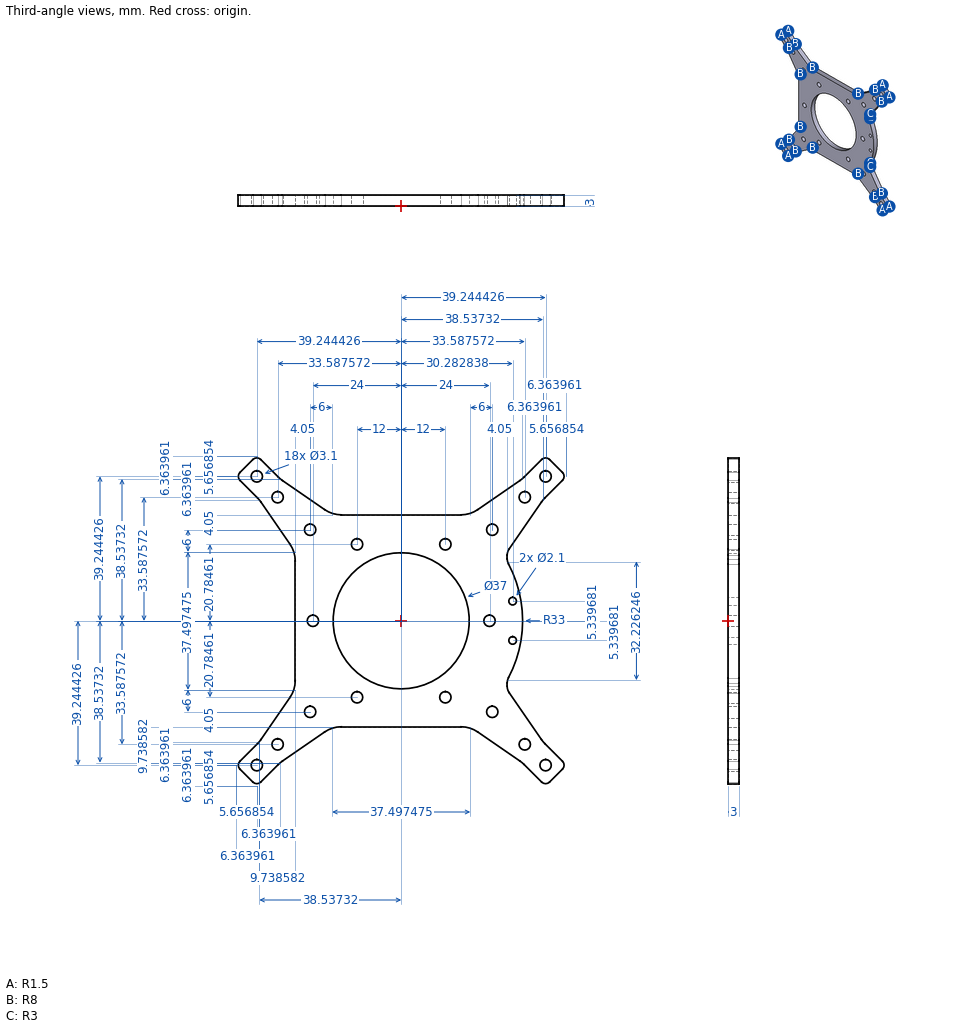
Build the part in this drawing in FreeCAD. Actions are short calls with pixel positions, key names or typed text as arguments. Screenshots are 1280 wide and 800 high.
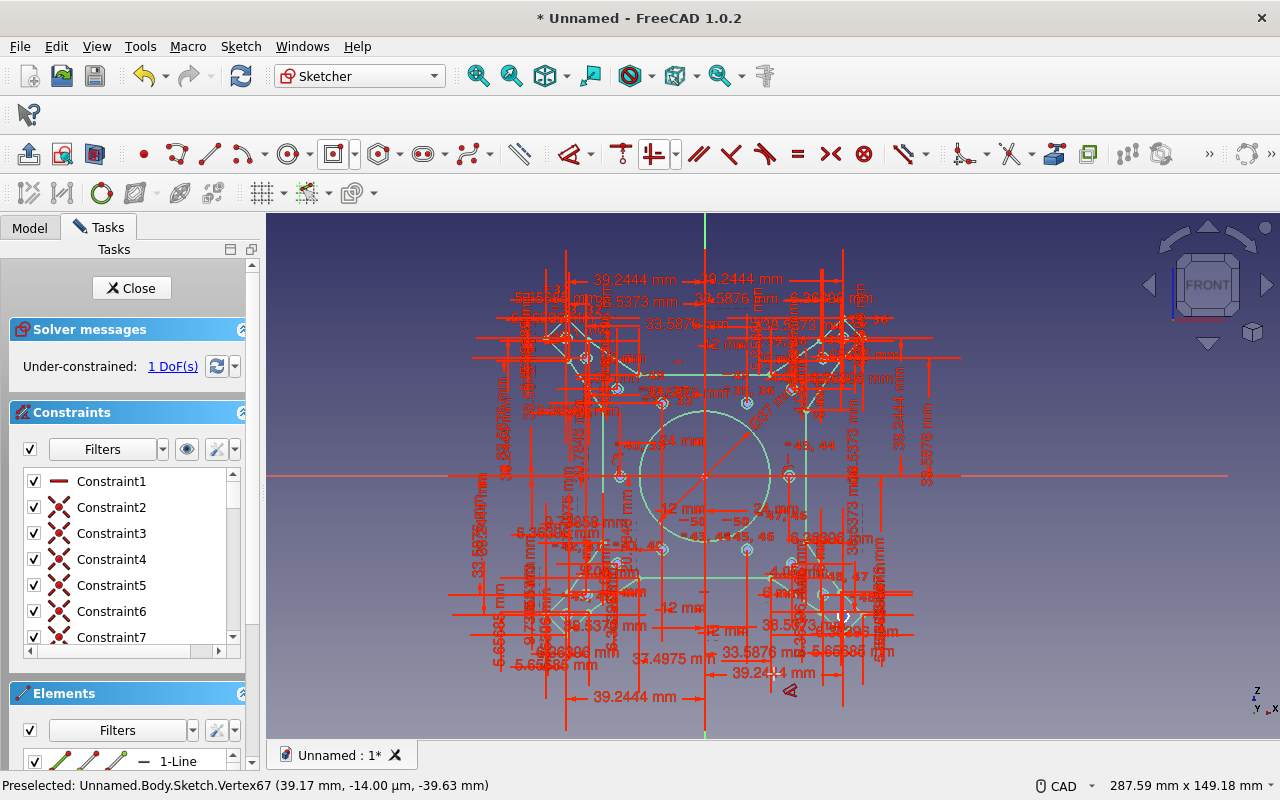
click(843, 616)
click(925, 546)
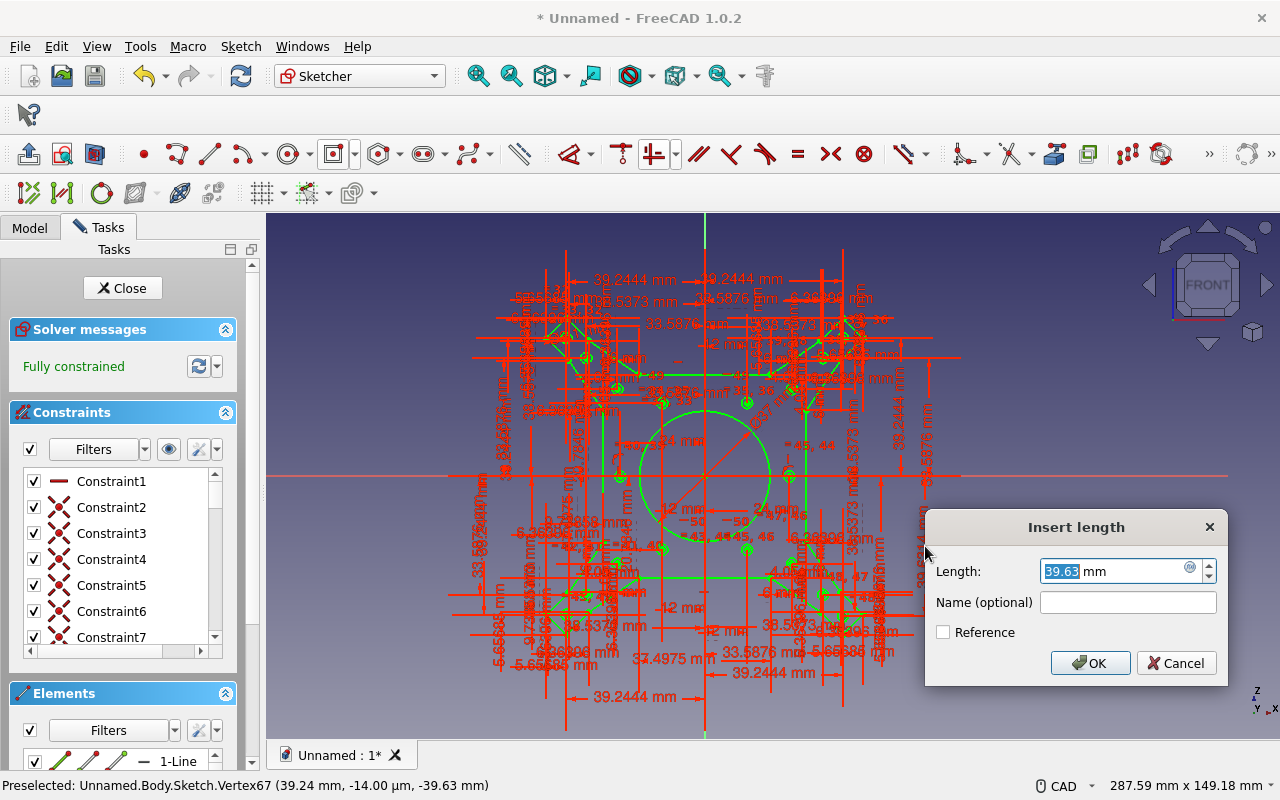
text(39.244426)
key(Return)
key(Escape)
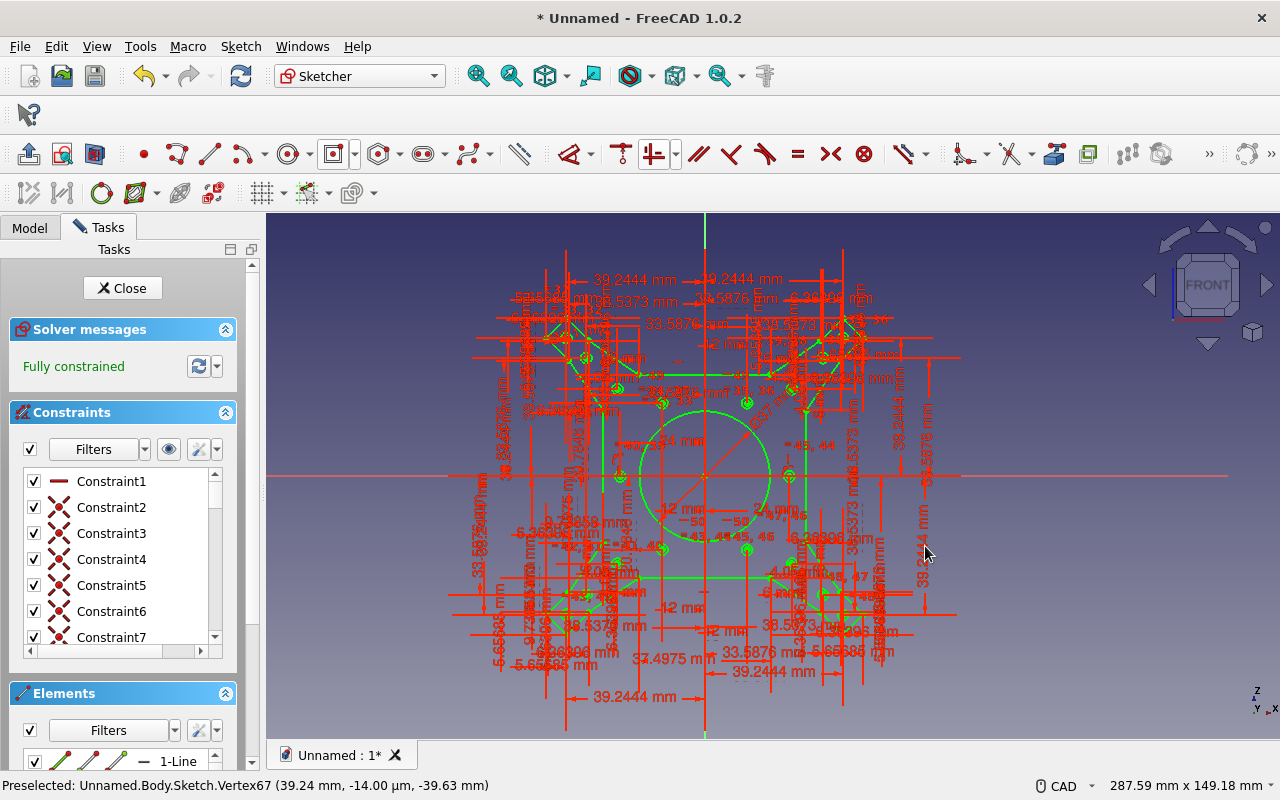
click(123, 288)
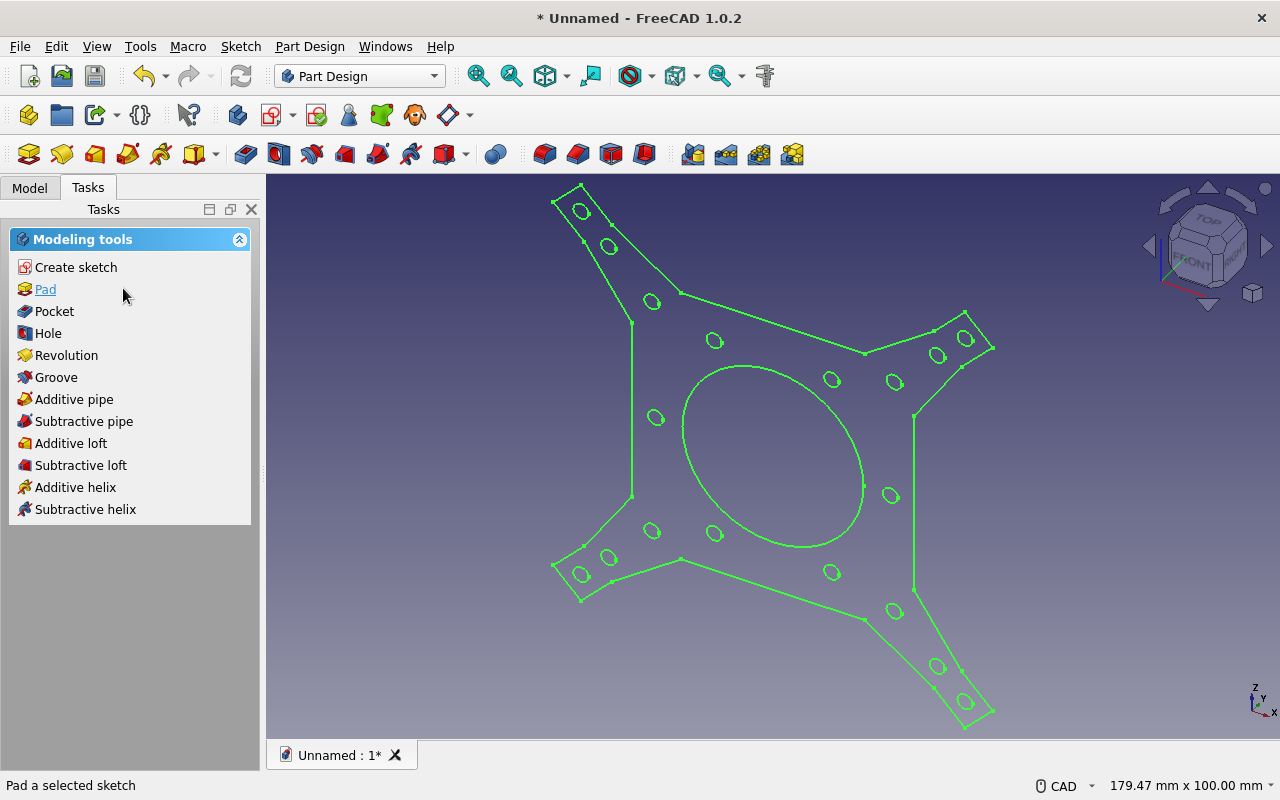
click(29, 154)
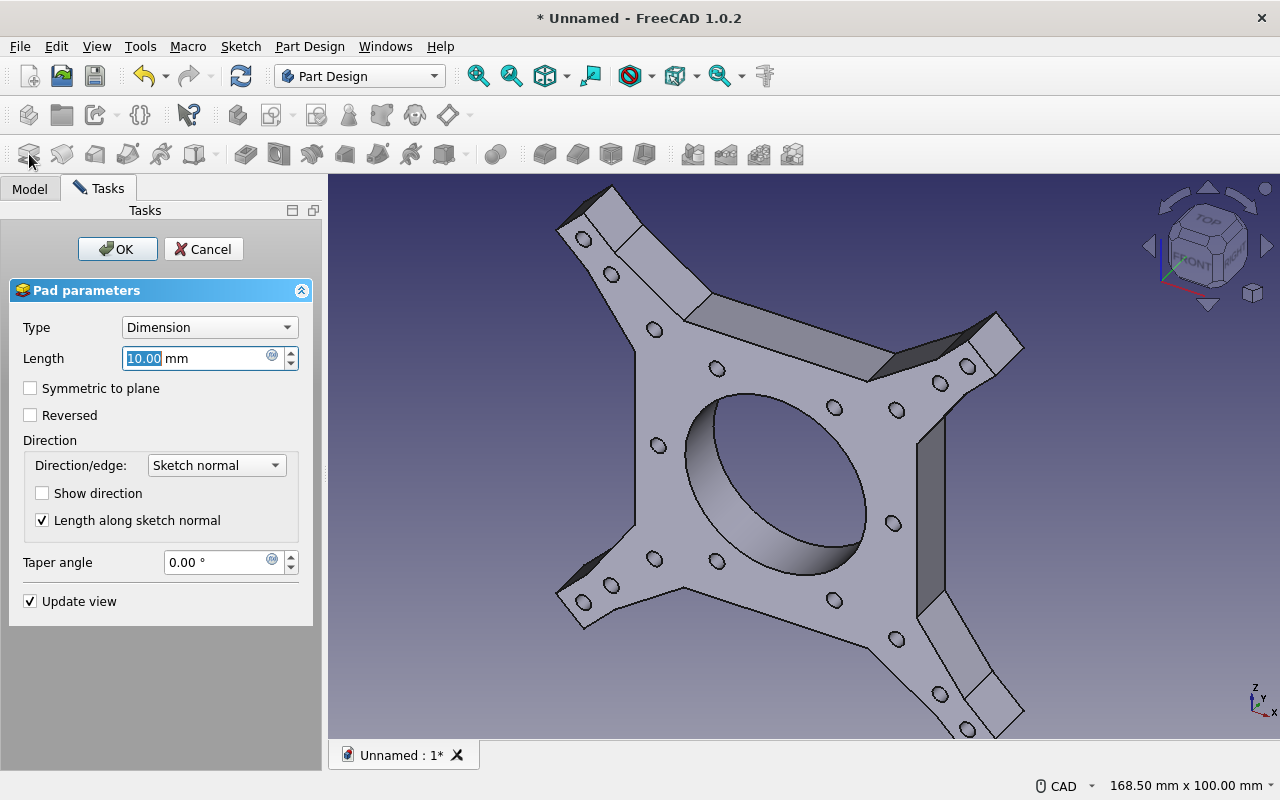
text(3)
key(Tab)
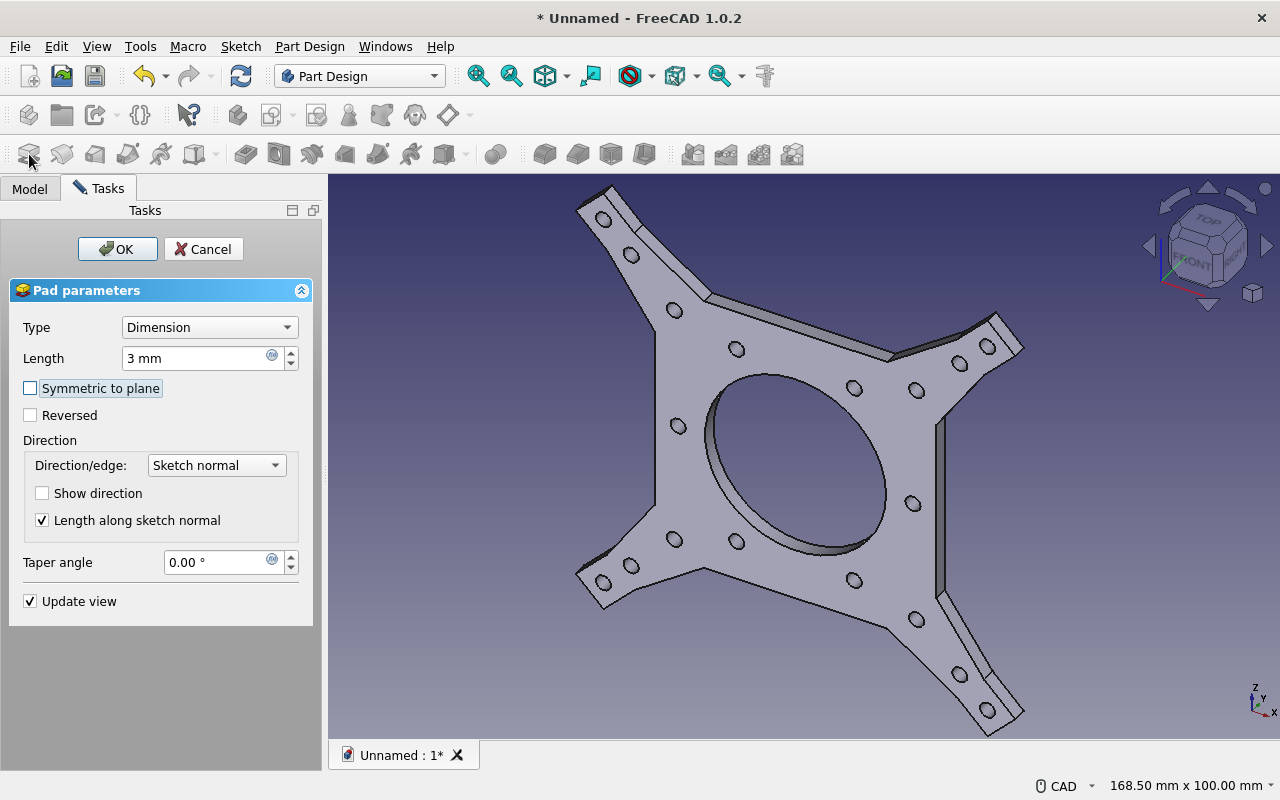
click(31, 415)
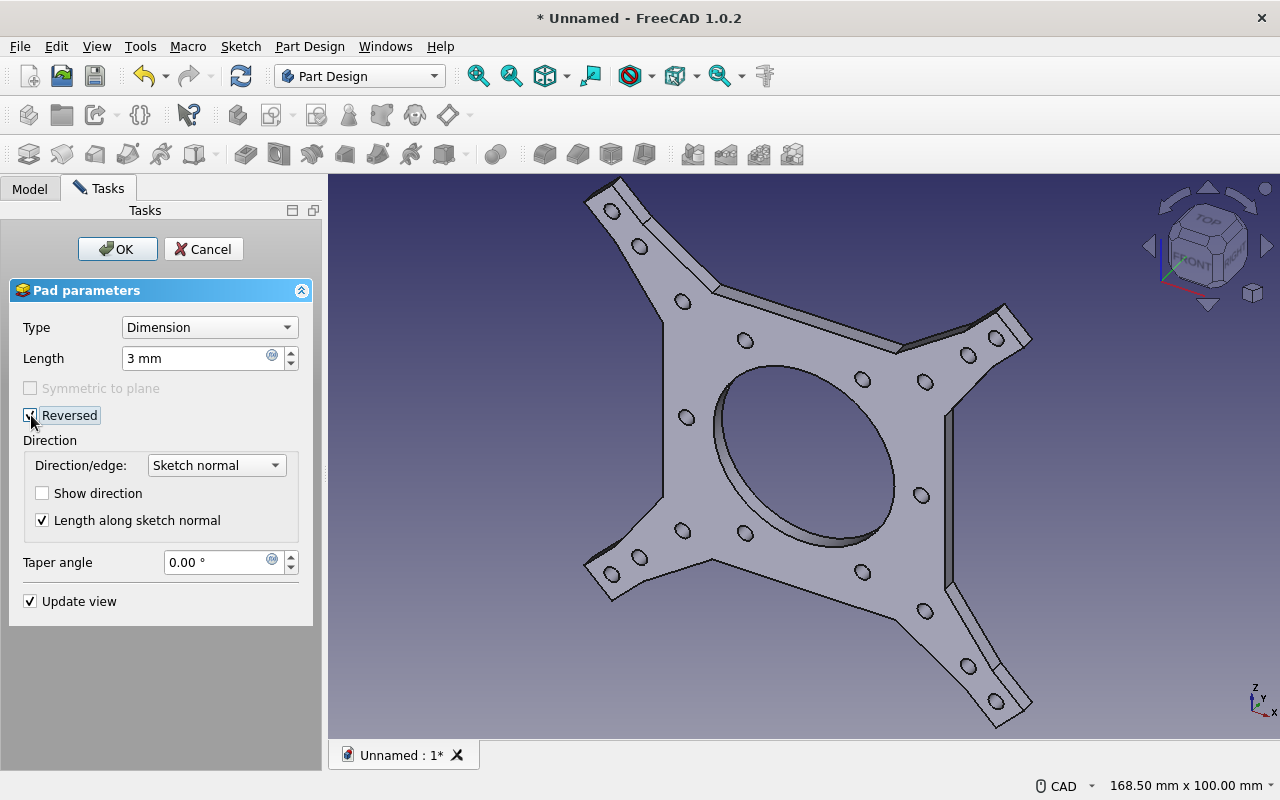
click(118, 249)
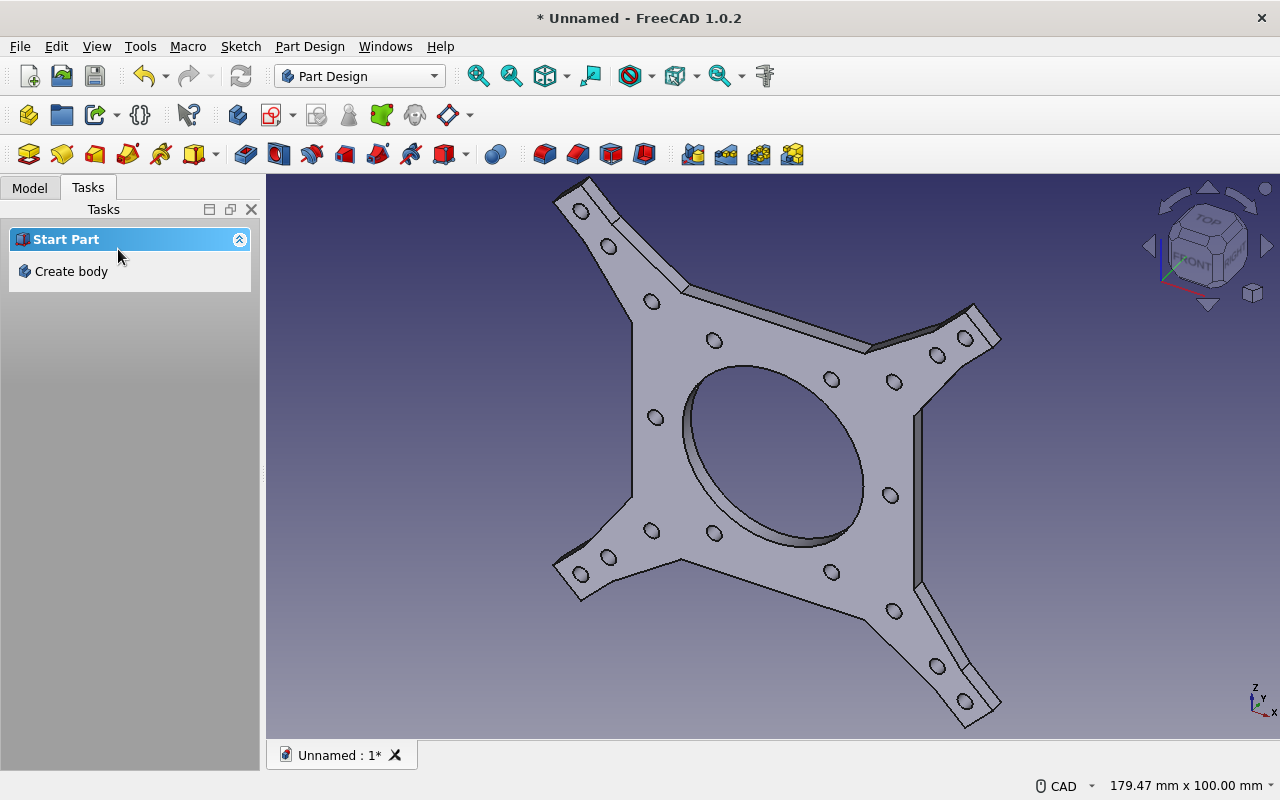
click(479, 76)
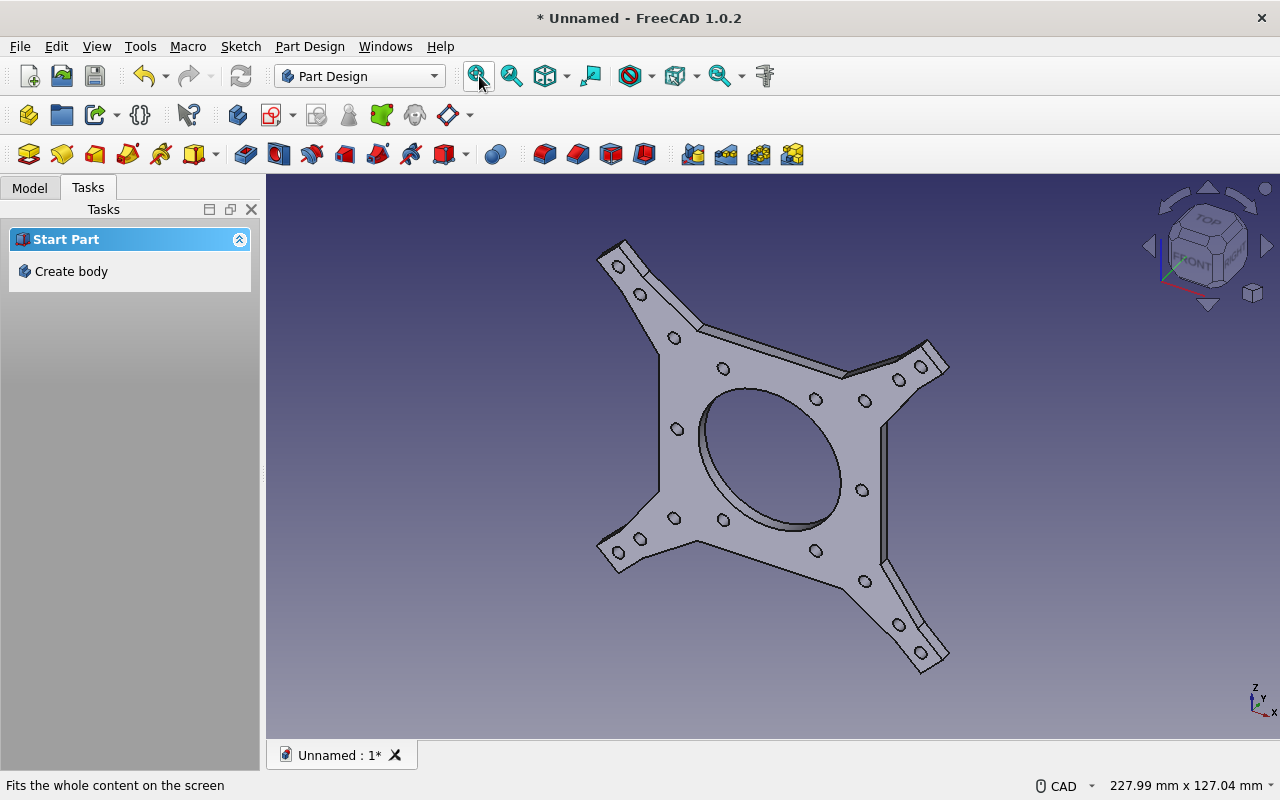
key(4)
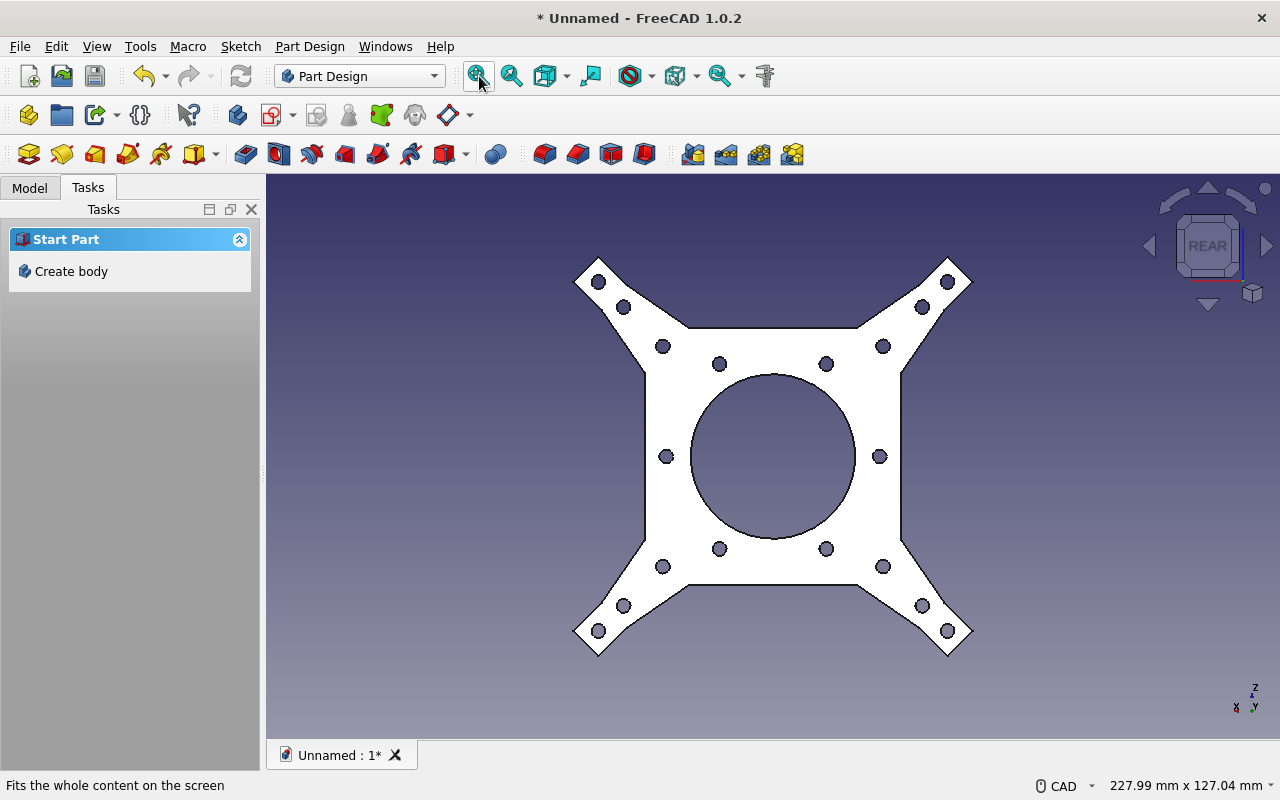
click(716, 570)